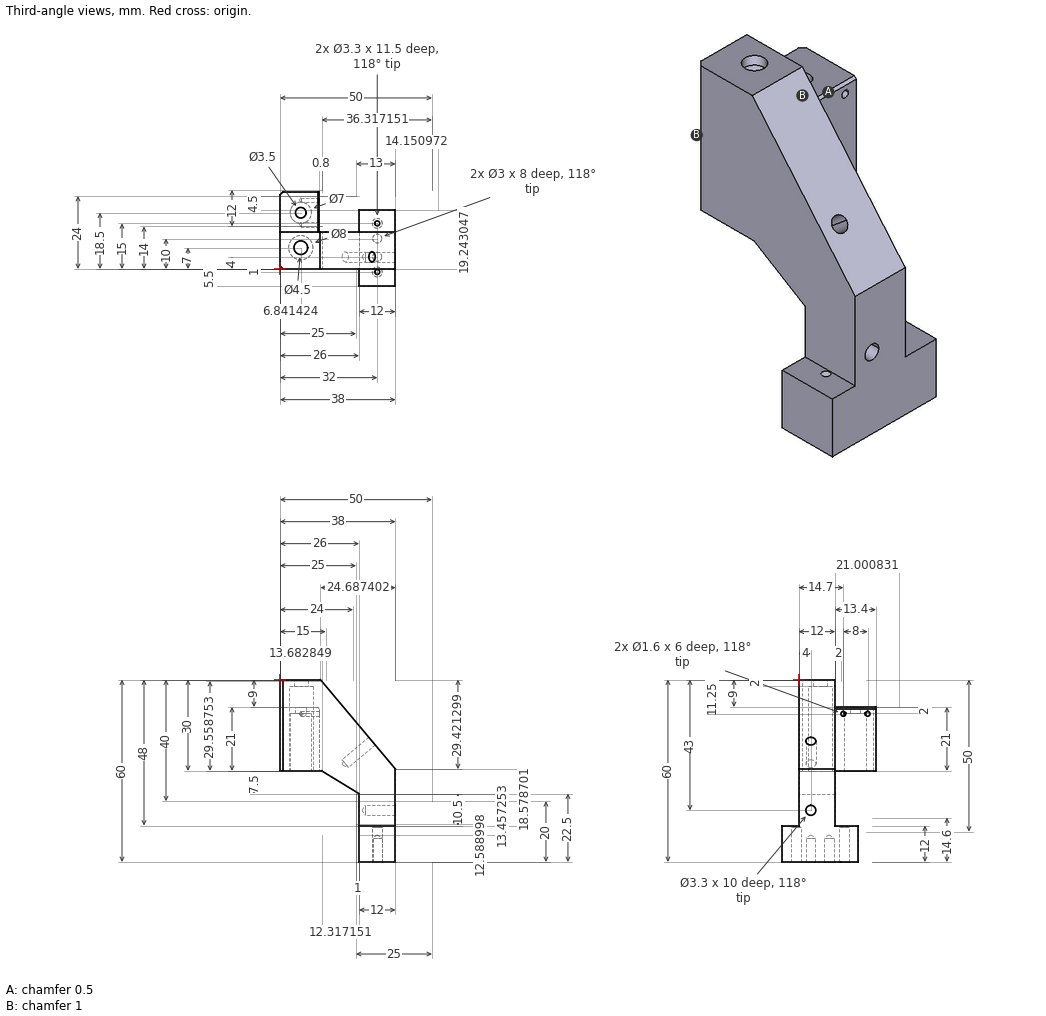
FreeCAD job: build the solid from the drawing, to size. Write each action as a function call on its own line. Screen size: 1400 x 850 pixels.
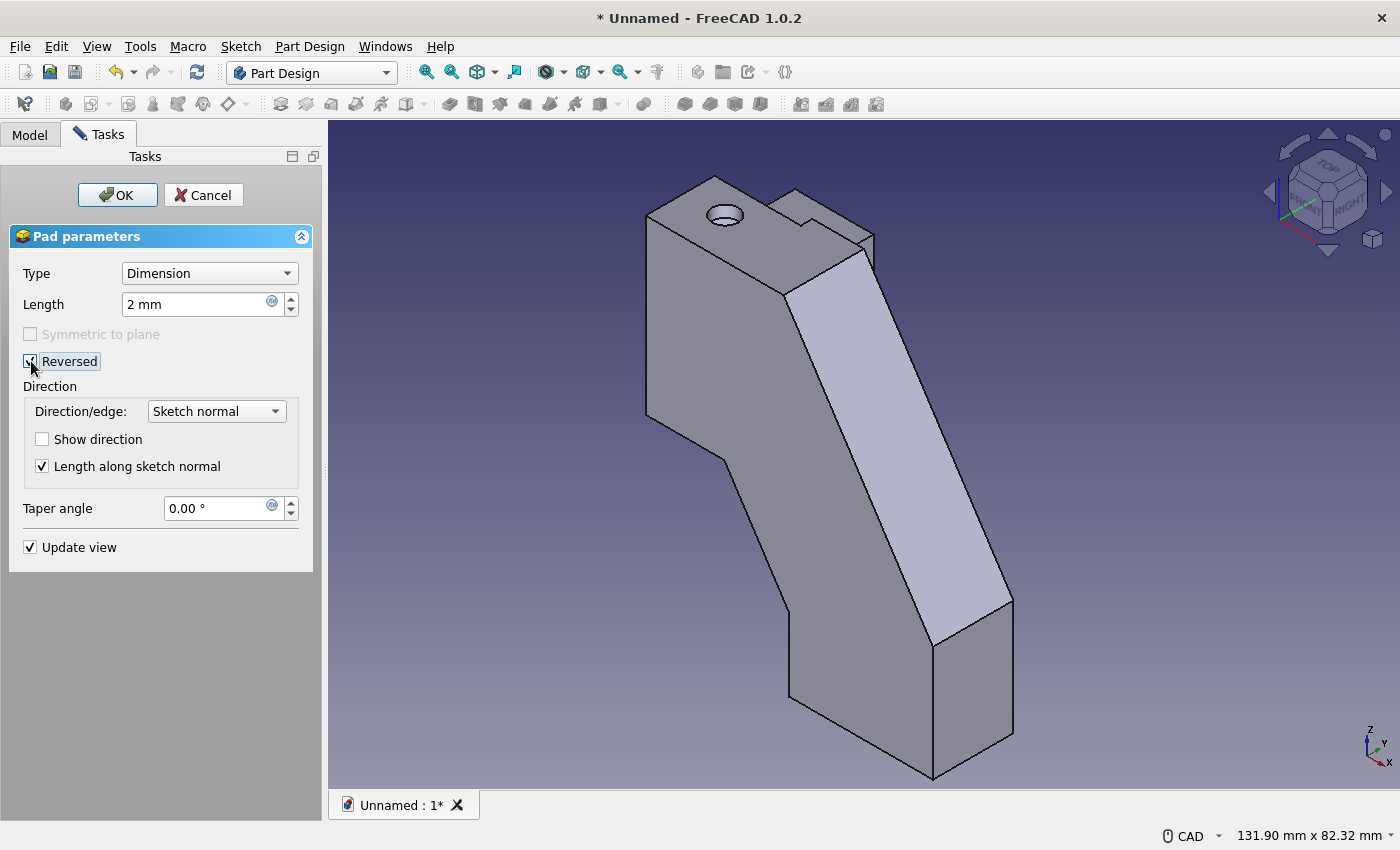
click(118, 195)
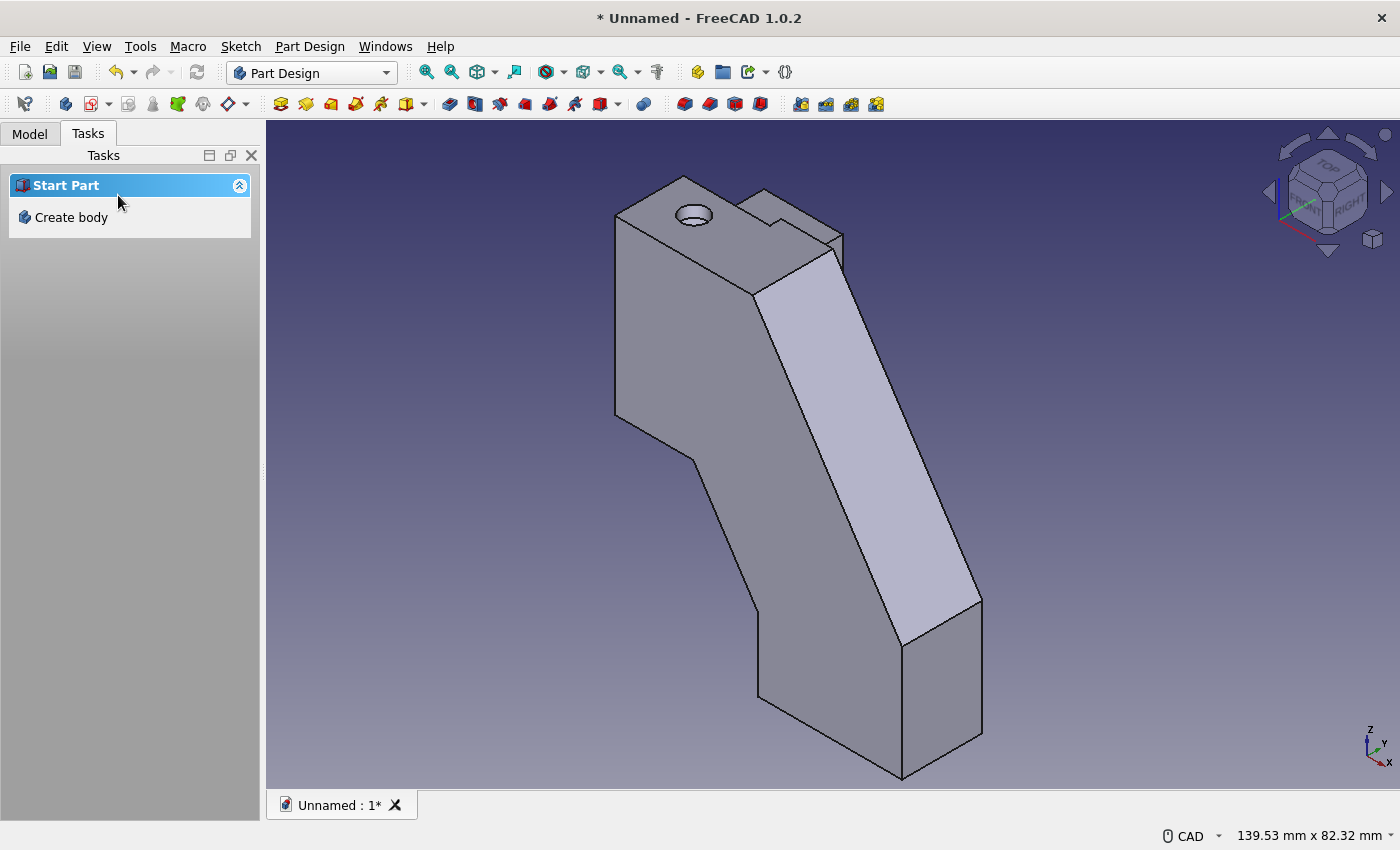
key(5)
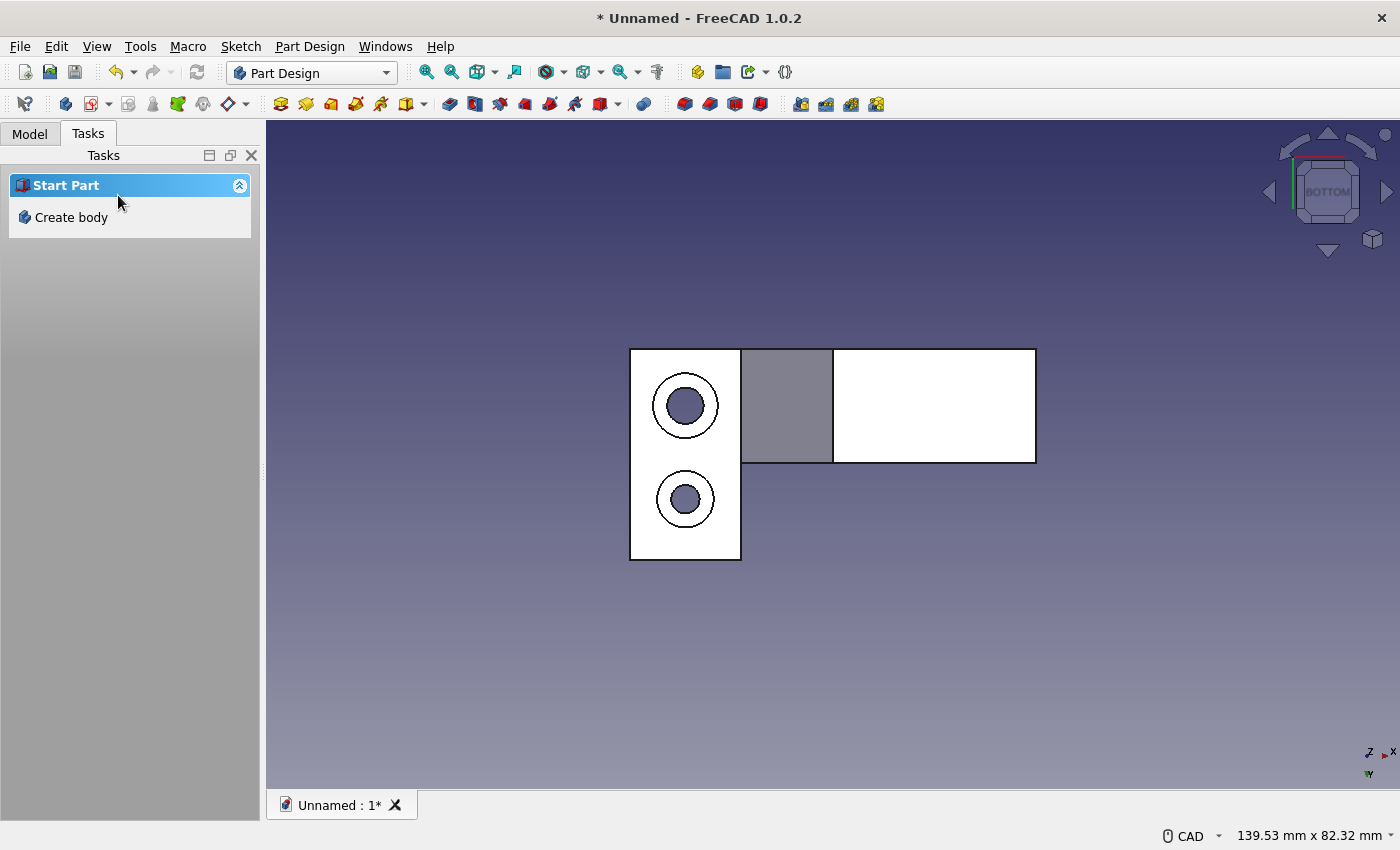
click(427, 72)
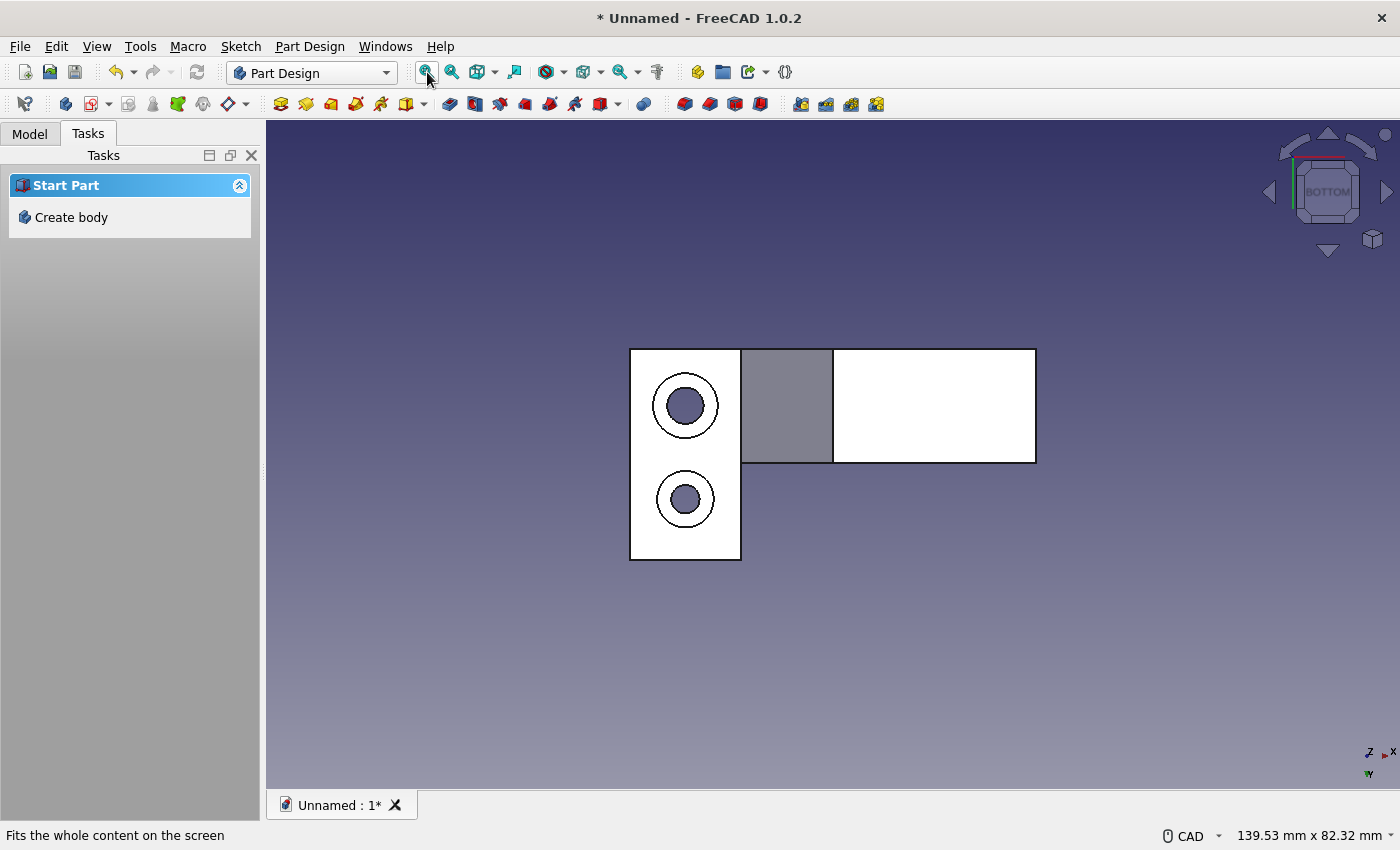
click(964, 405)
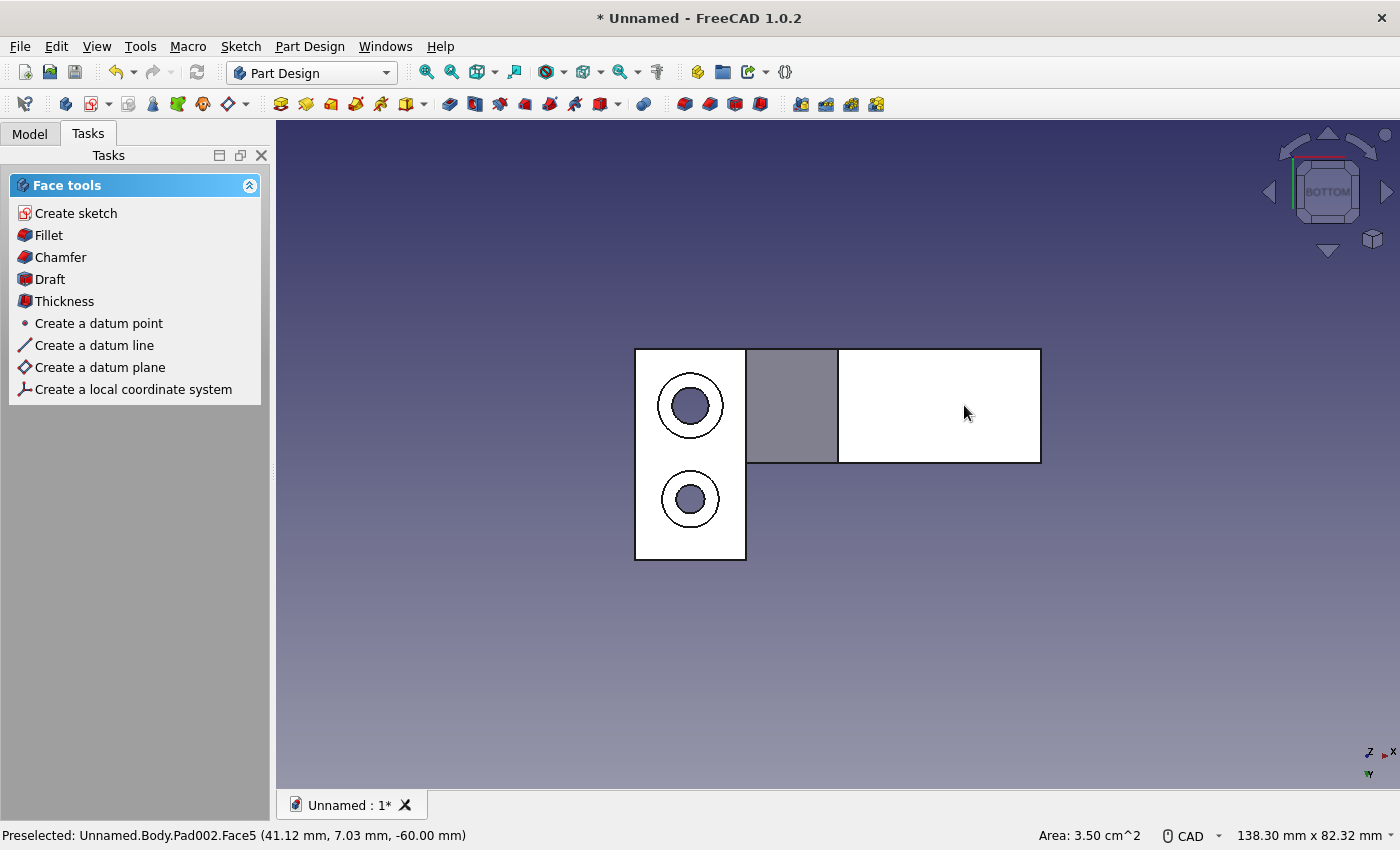
click(90, 104)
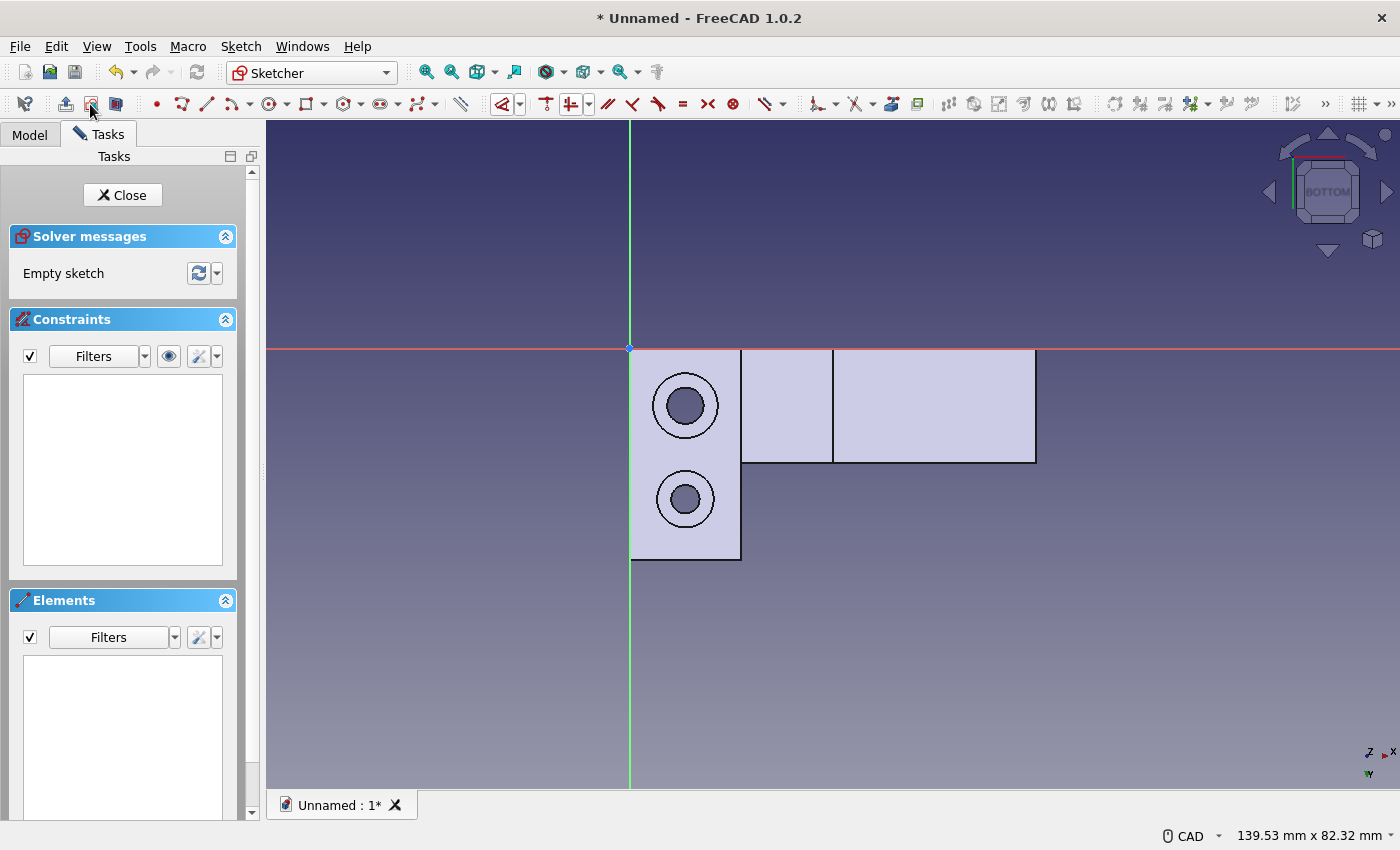
scroll(1131, 411, up, 5)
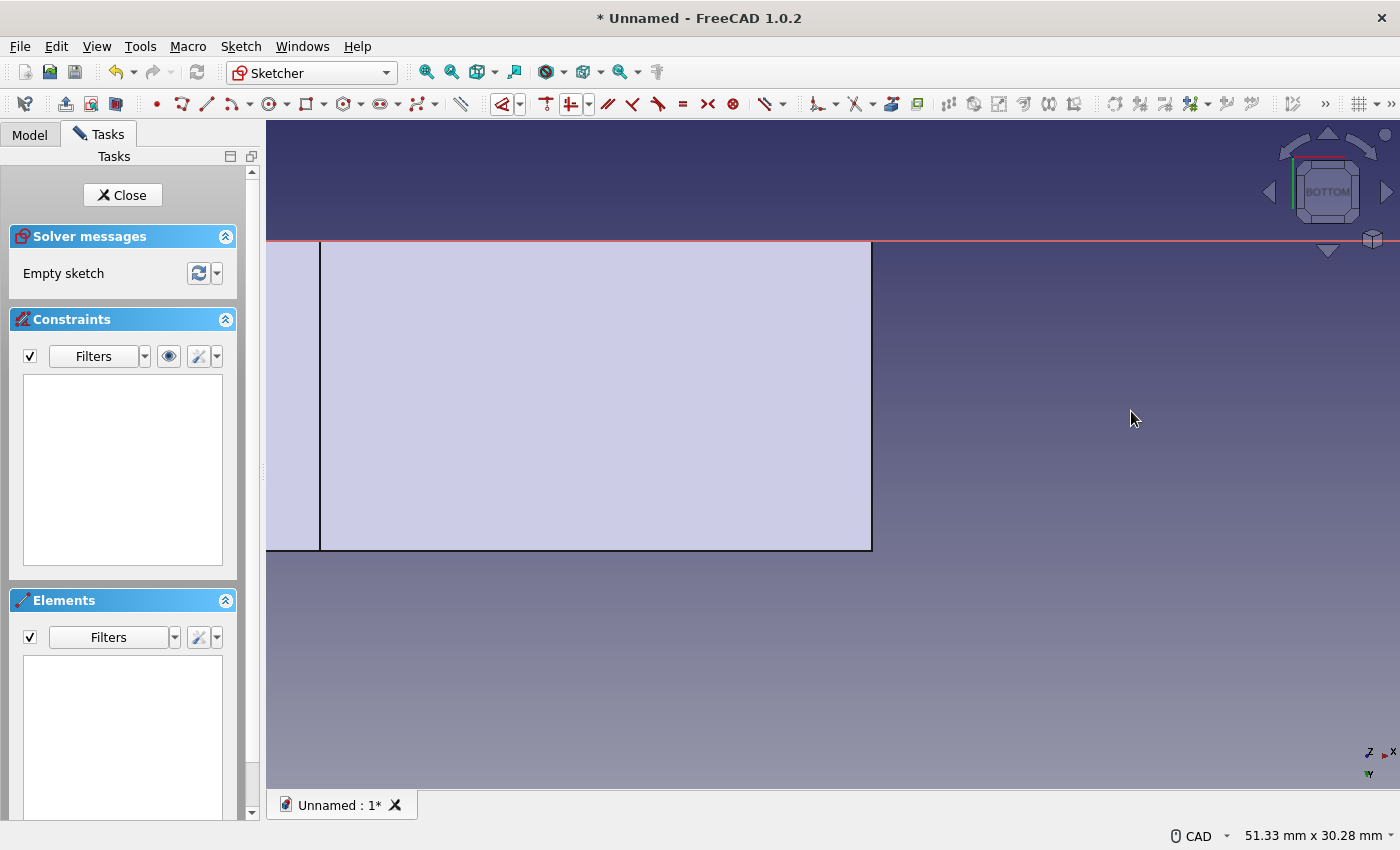
click(306, 104)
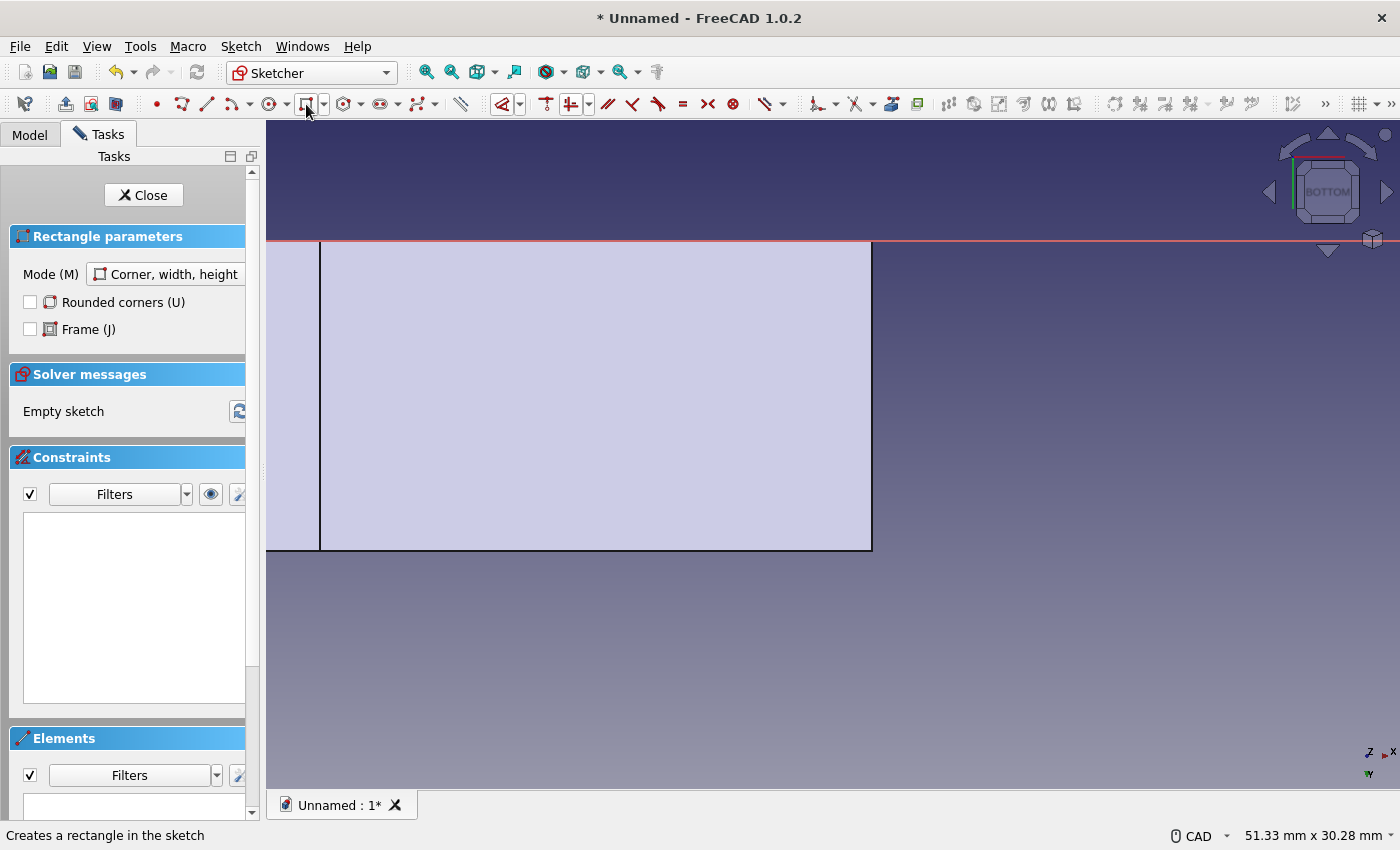
click(607, 241)
click(919, 666)
key(Escape)